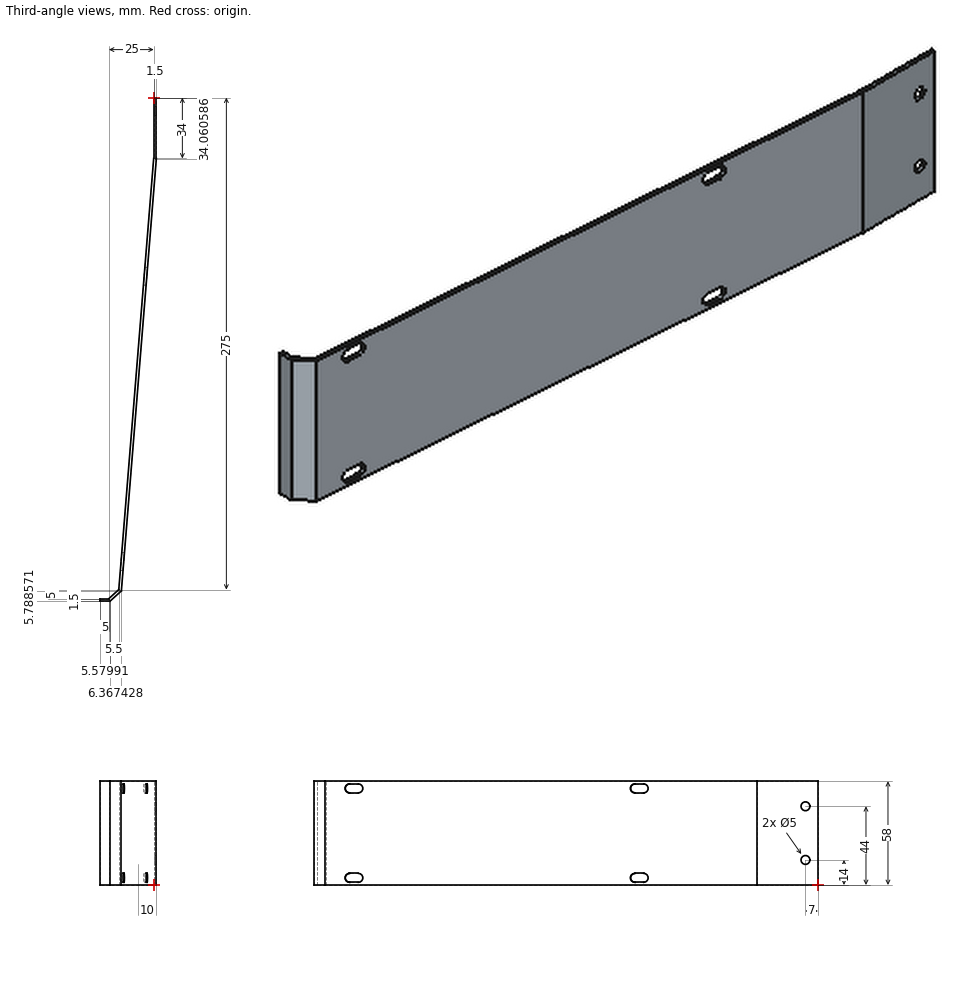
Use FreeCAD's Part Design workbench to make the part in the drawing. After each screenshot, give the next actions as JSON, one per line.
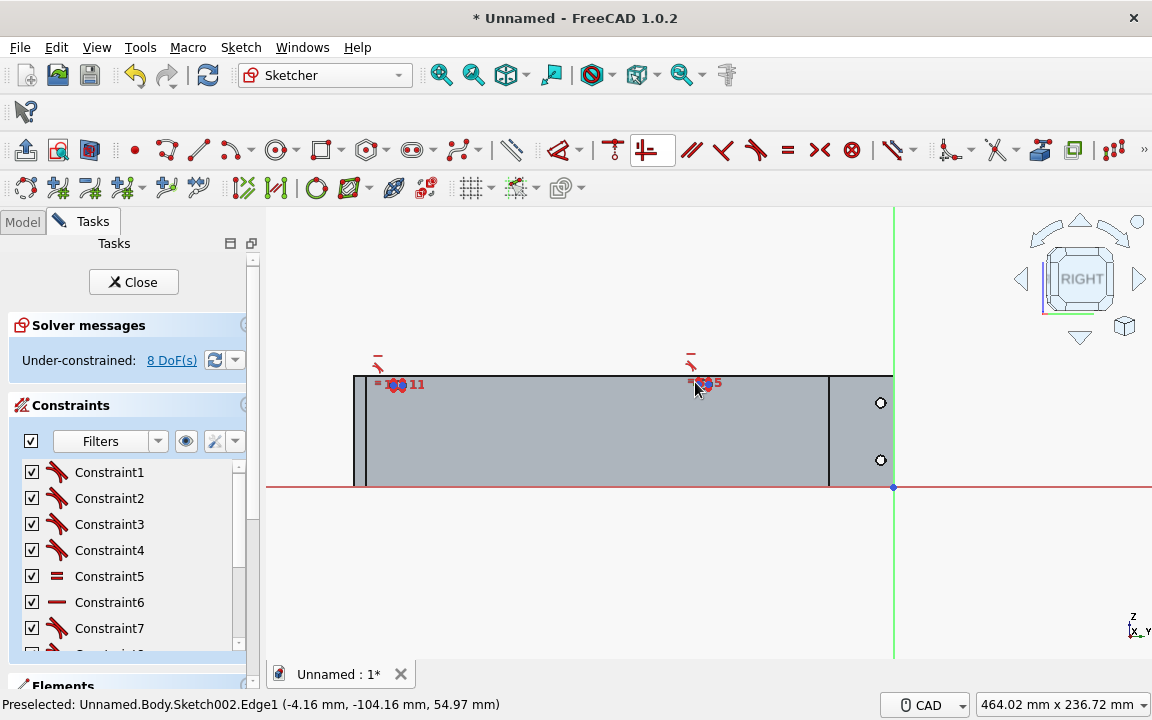
{"action": "scroll", "coordinate": [390, 383], "scroll_direction": "up", "scroll_amount": 7}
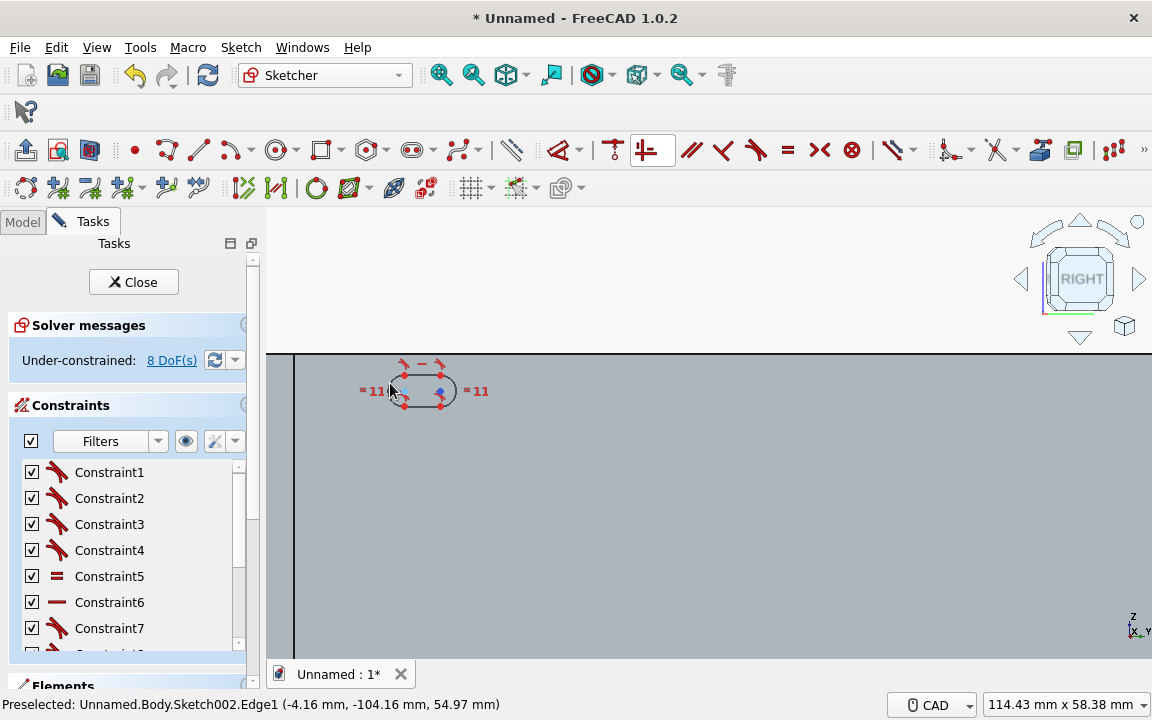
{"action": "left_click", "coordinate": [391, 382]}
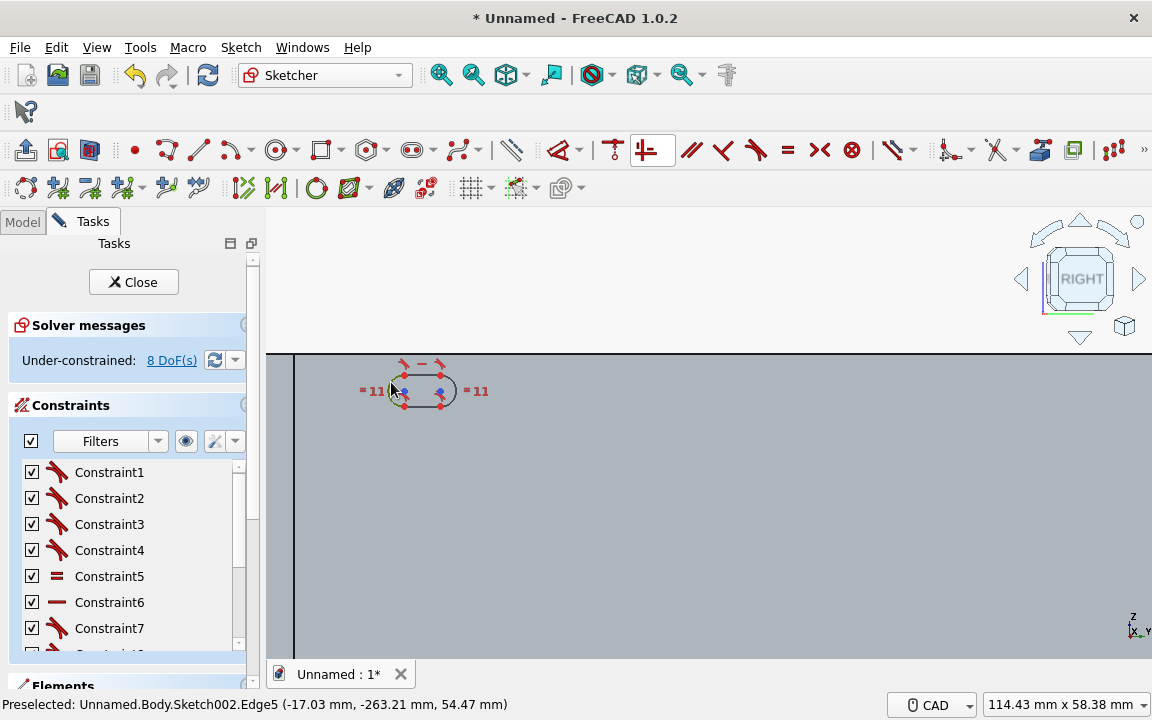
{"action": "left_click", "coordinate": [788, 150]}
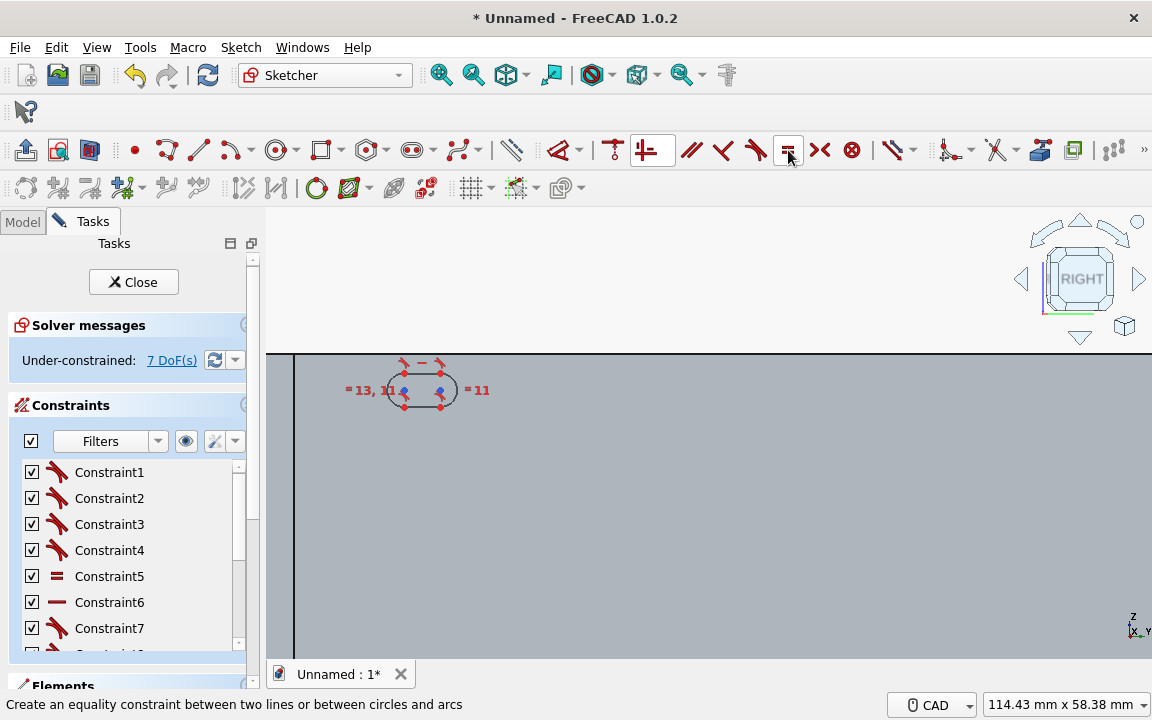
{"action": "left_click", "coordinate": [558, 150]}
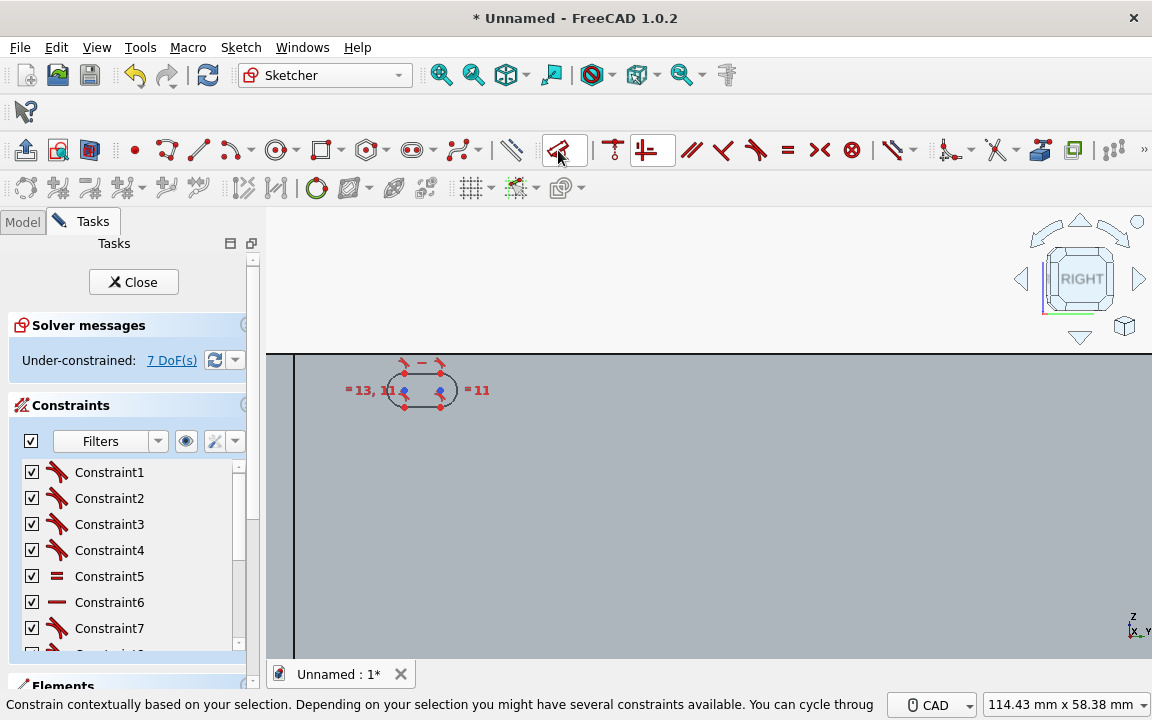
{"action": "scroll", "coordinate": [389, 383], "scroll_direction": "down", "scroll_amount": 7}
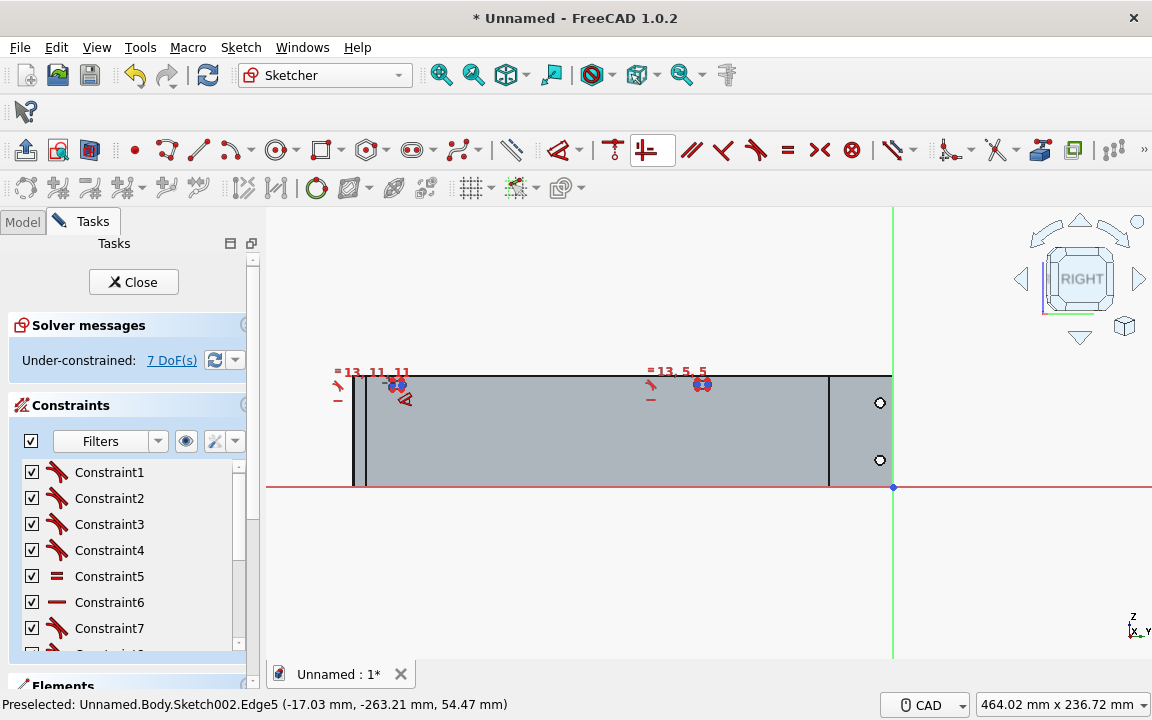
{"action": "scroll", "coordinate": [695, 382], "scroll_direction": "up", "scroll_amount": 11}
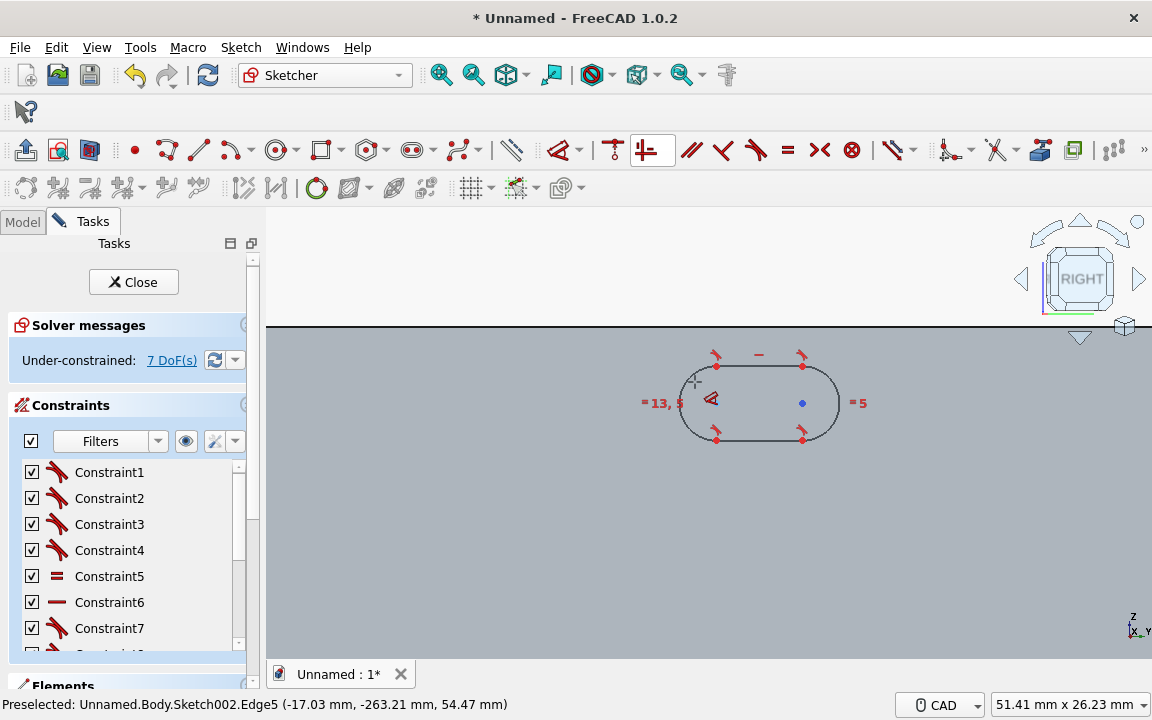
{"action": "left_click", "coordinate": [687, 382]}
{"action": "left_click", "coordinate": [661, 363]}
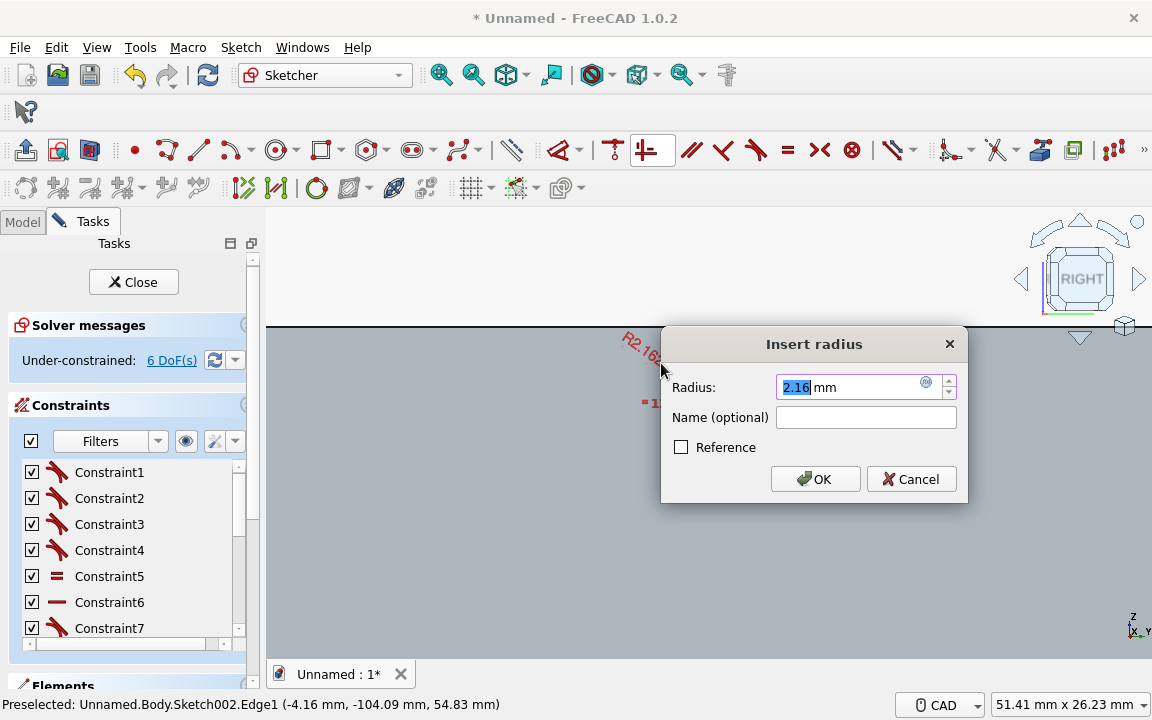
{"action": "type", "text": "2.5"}
{"action": "key", "text": "Return"}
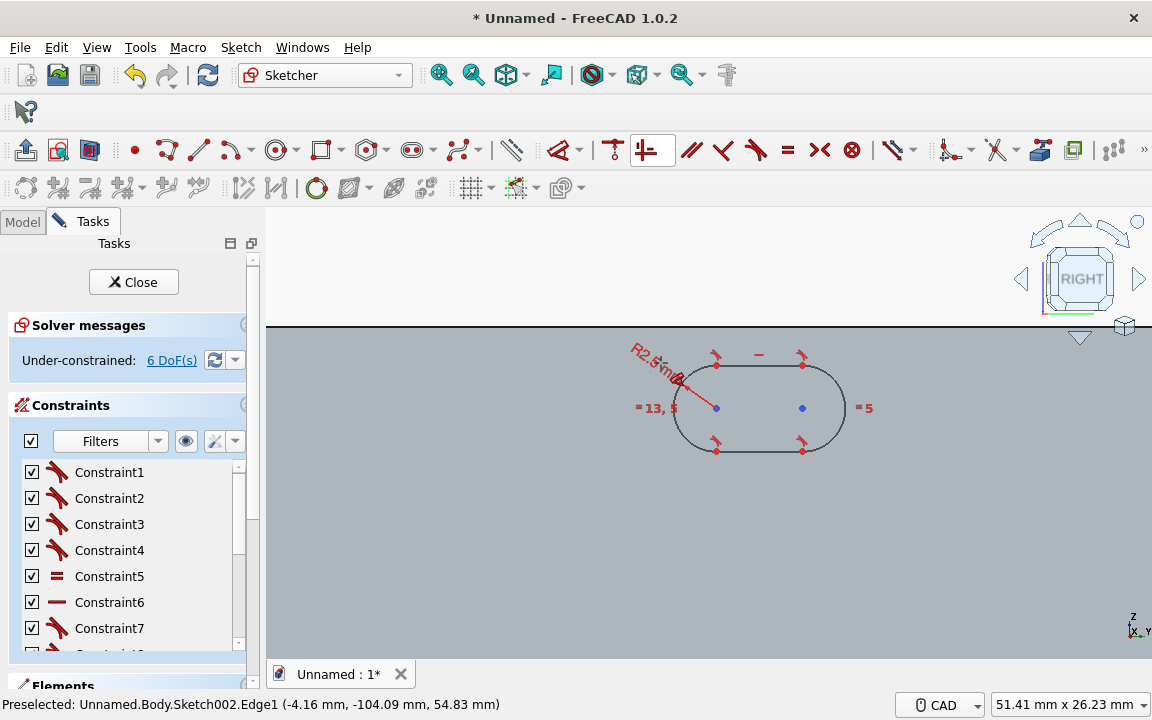
{"action": "left_click", "coordinate": [742, 366]}
{"action": "left_click", "coordinate": [759, 332]}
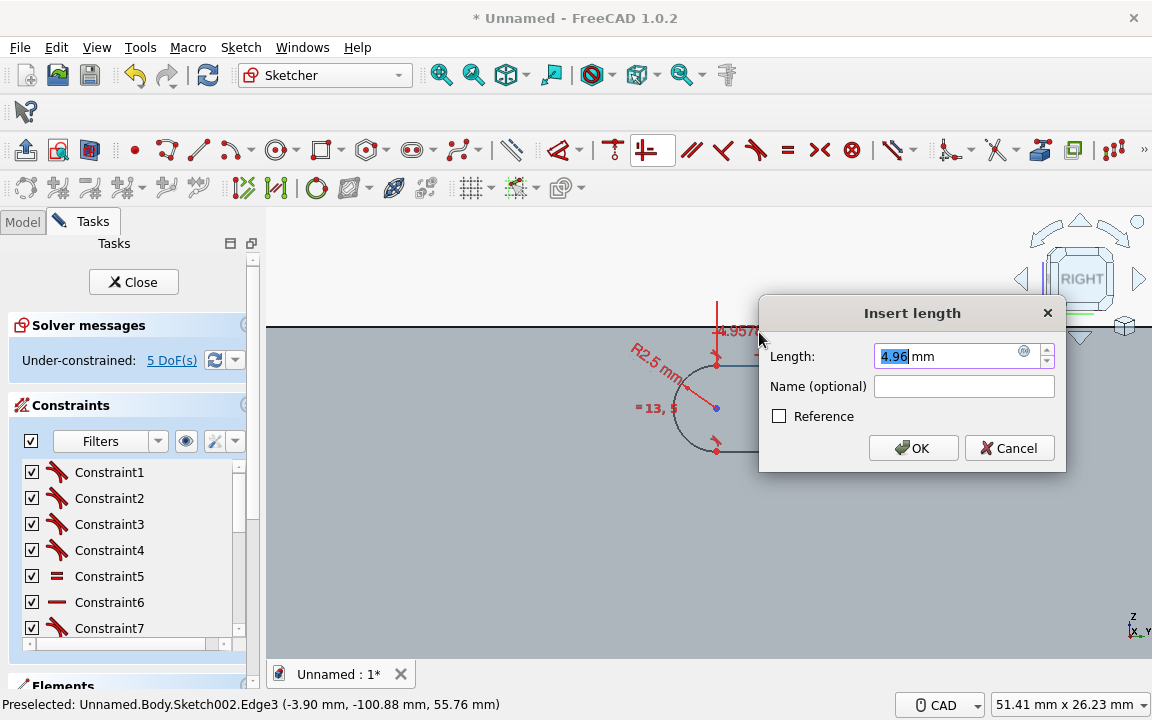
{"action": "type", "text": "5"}
{"action": "key", "text": "Return"}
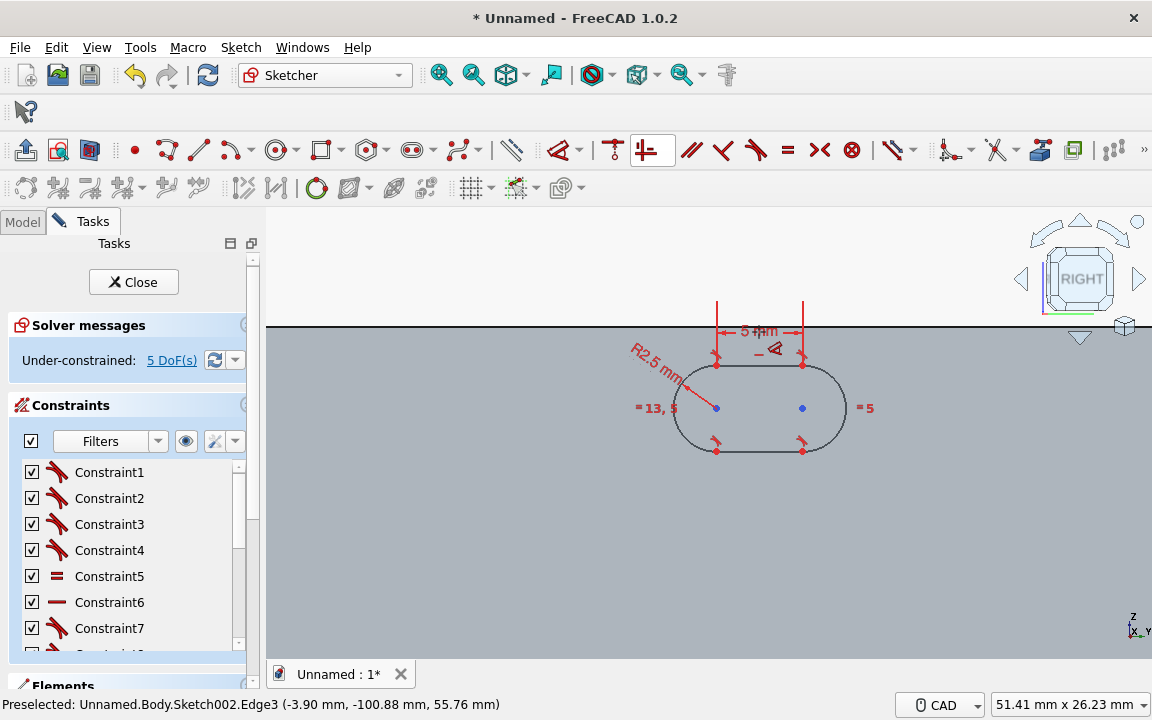
{"action": "scroll", "coordinate": [696, 382], "scroll_direction": "down", "scroll_amount": 11}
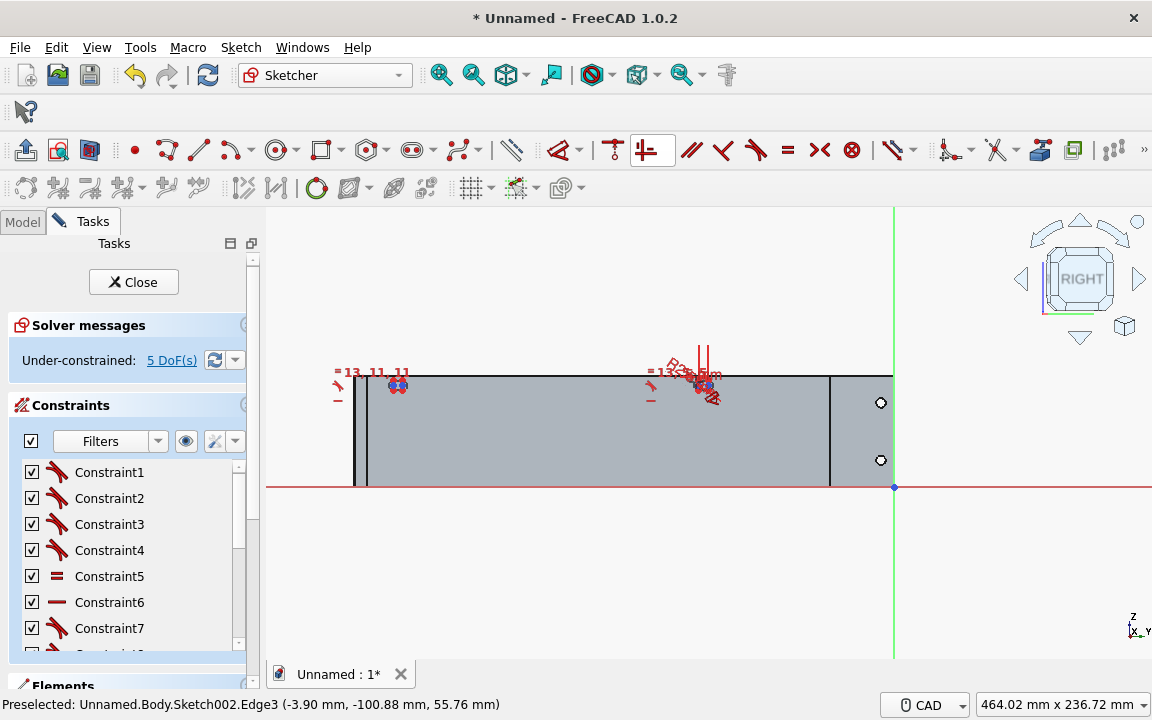
{"action": "scroll", "coordinate": [396, 381], "scroll_direction": "up", "scroll_amount": 9}